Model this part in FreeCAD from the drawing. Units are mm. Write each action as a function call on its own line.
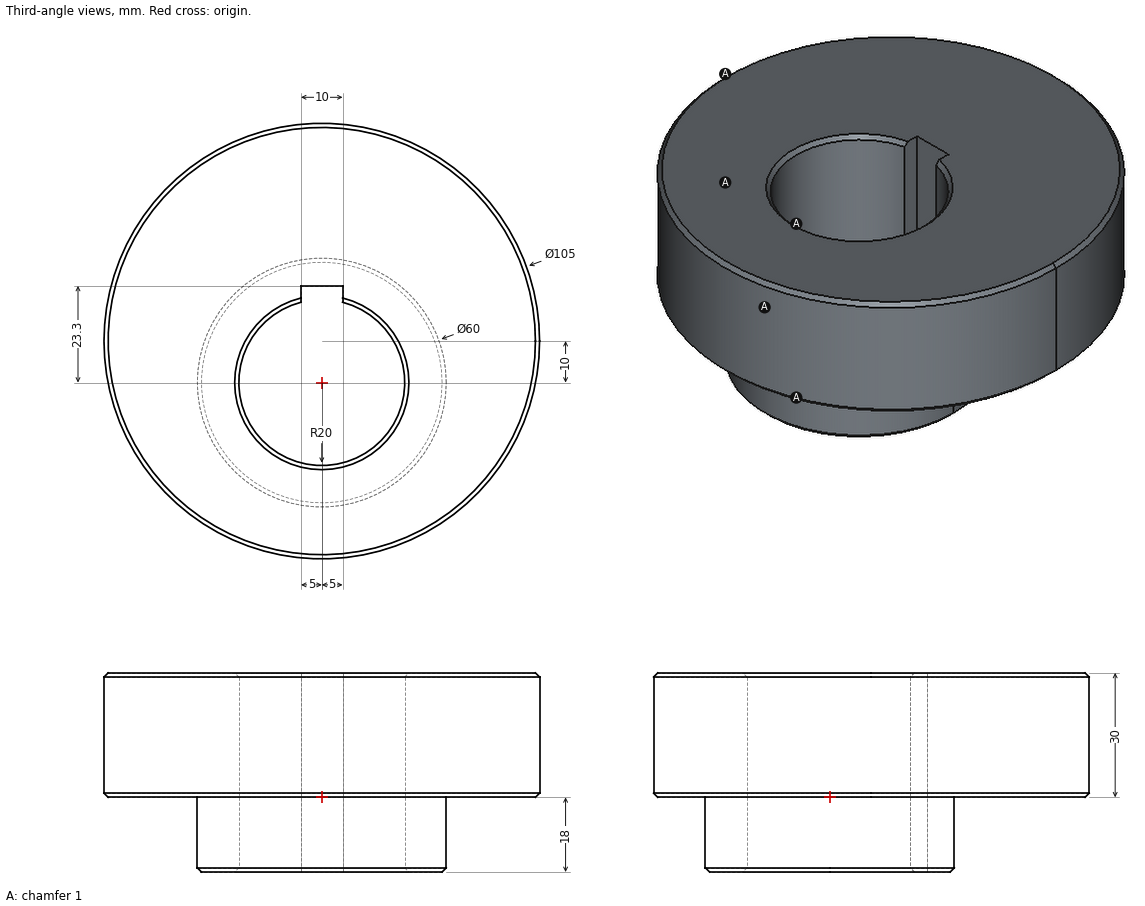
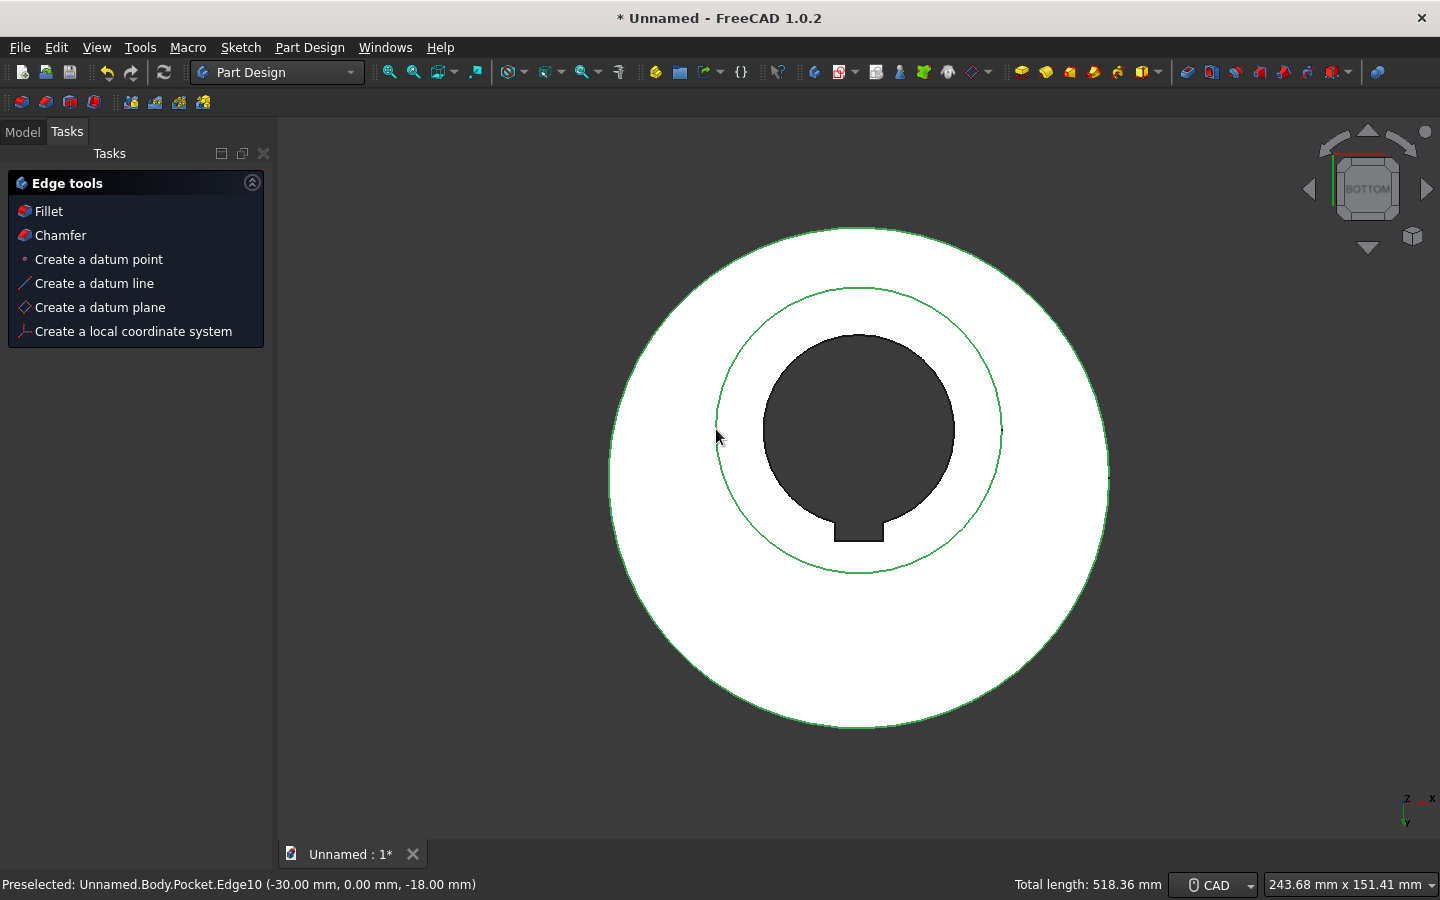
click(859, 334, ctrl)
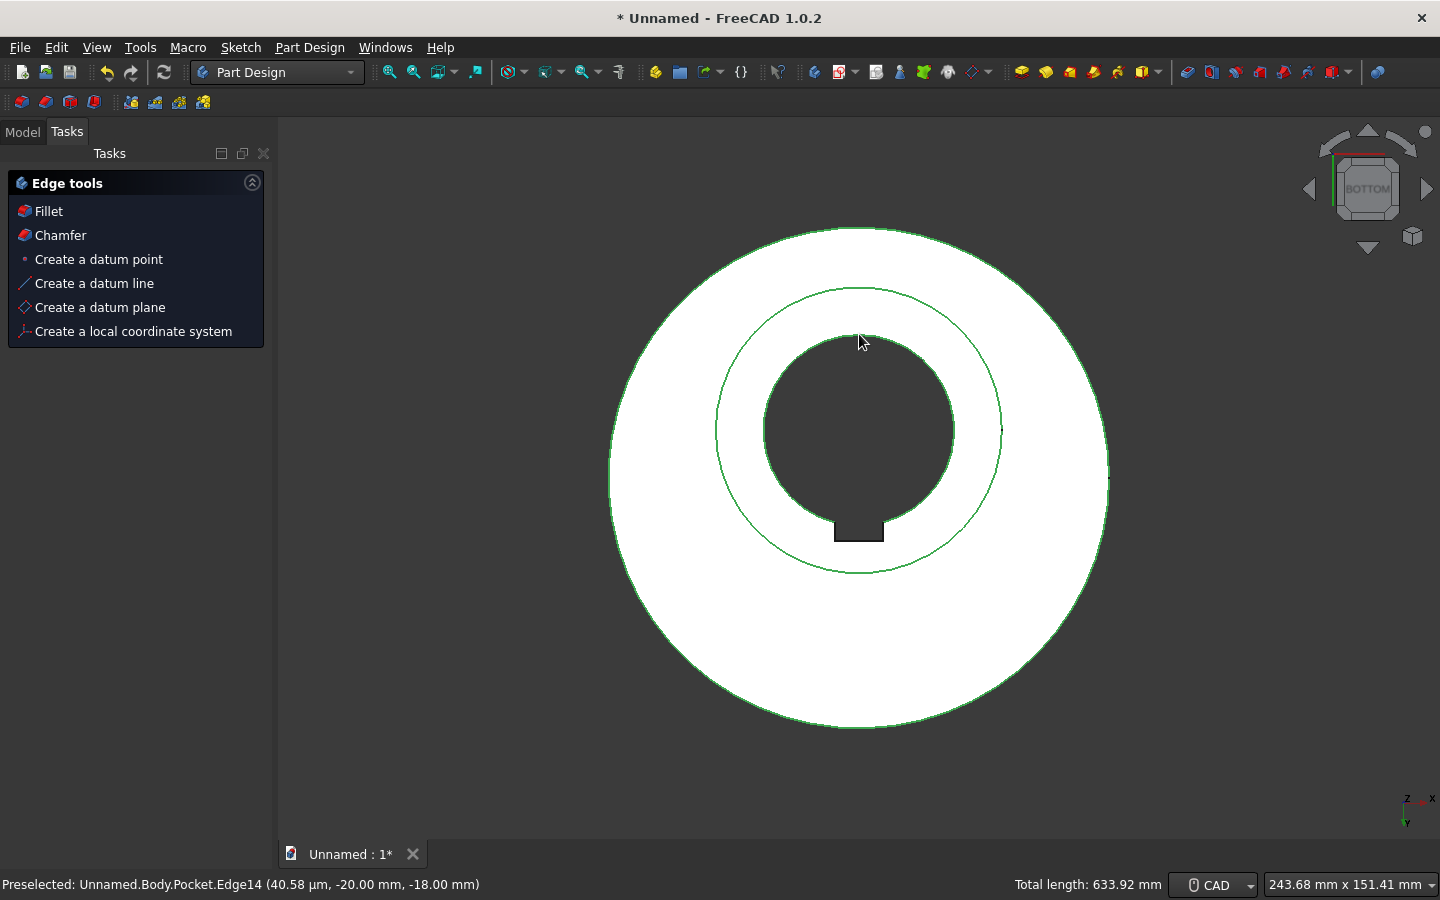
key(0)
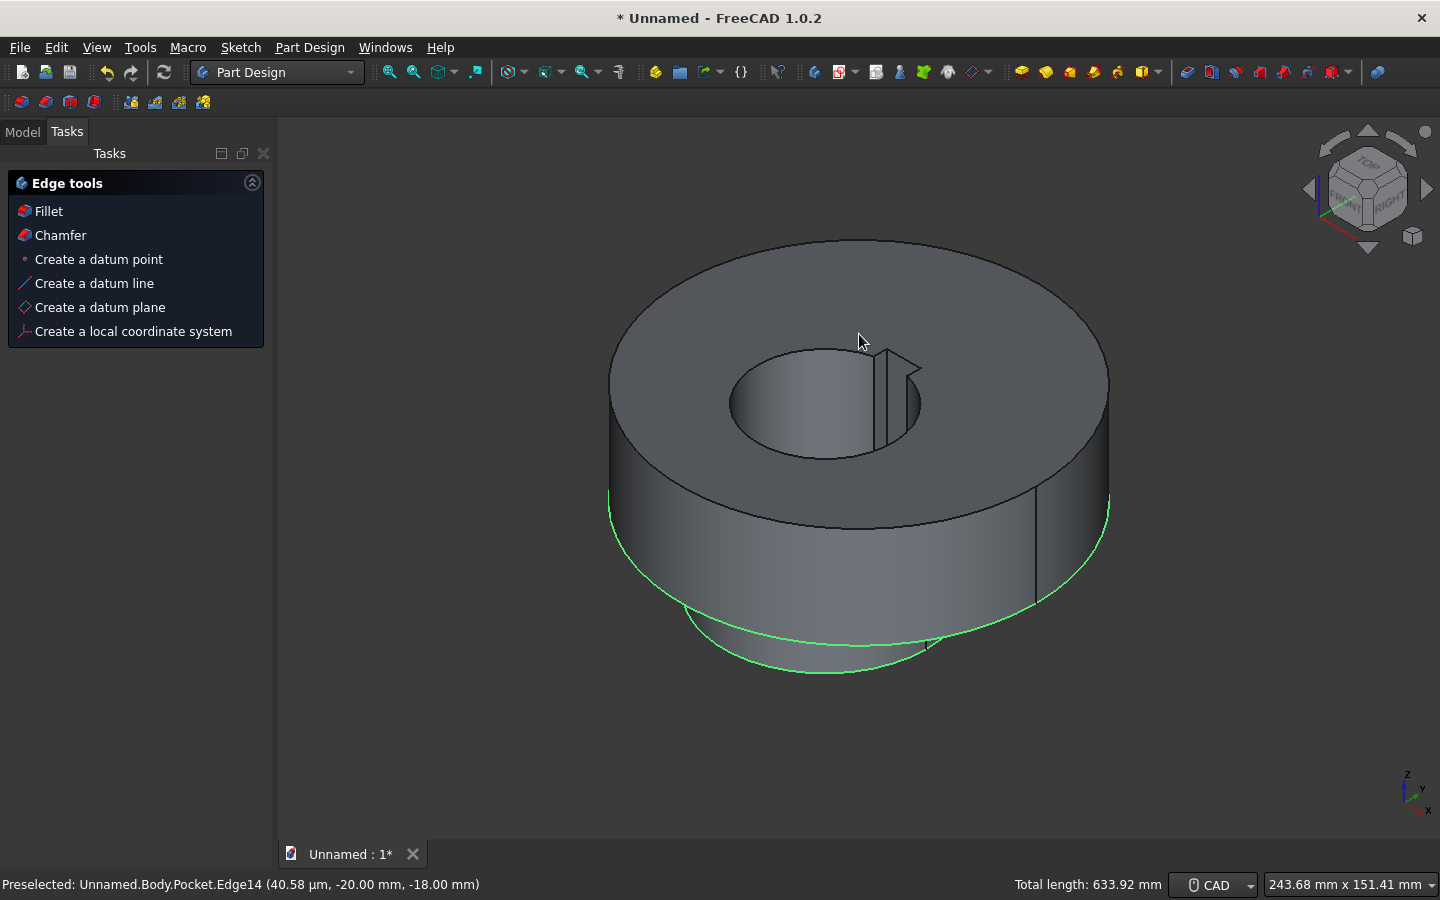
click(736, 383, ctrl)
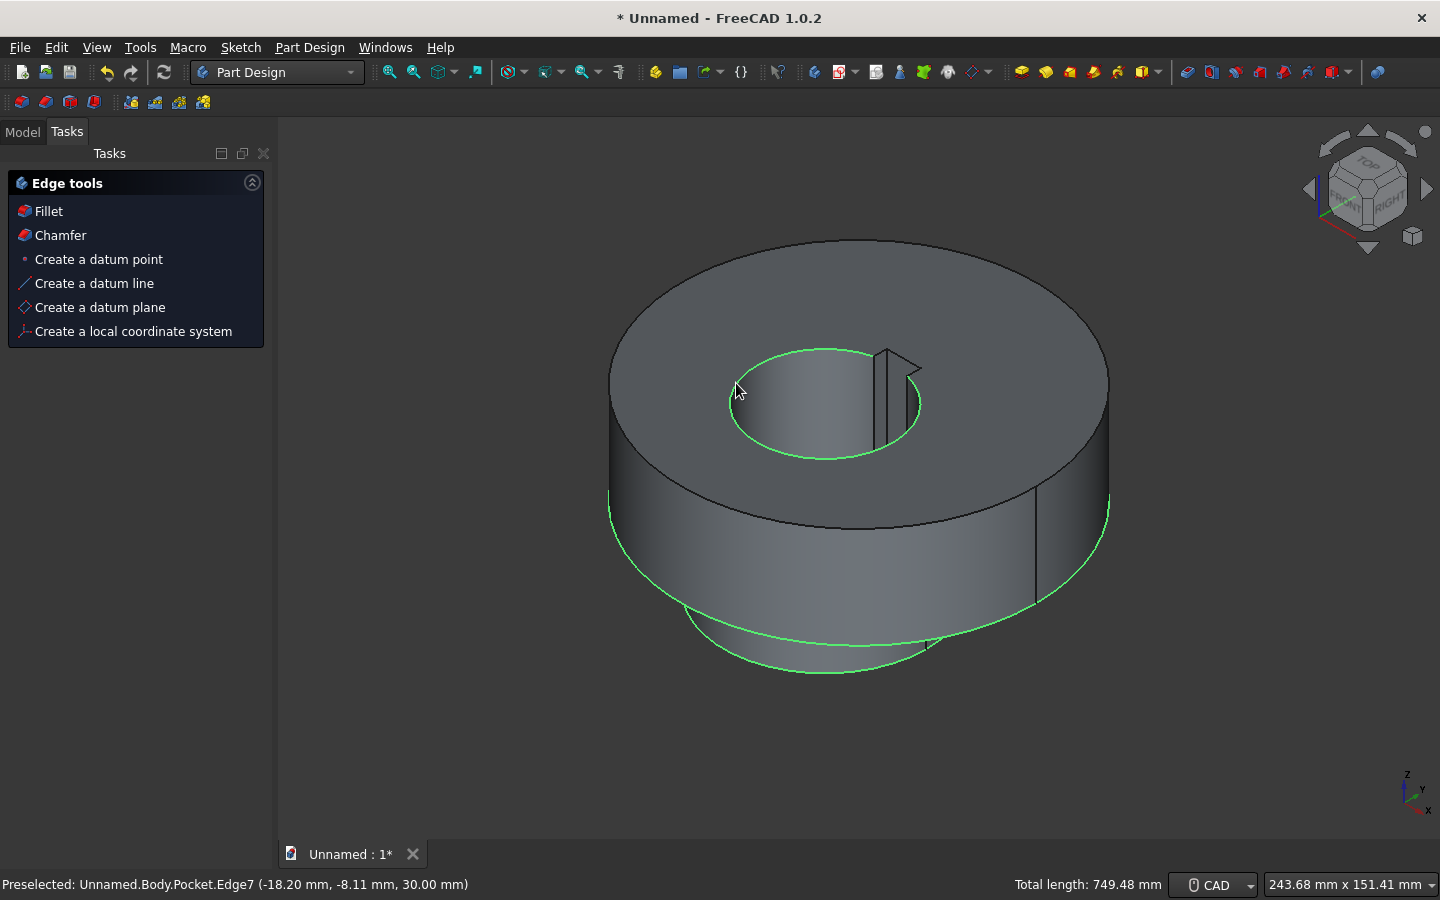
click(636, 449, ctrl)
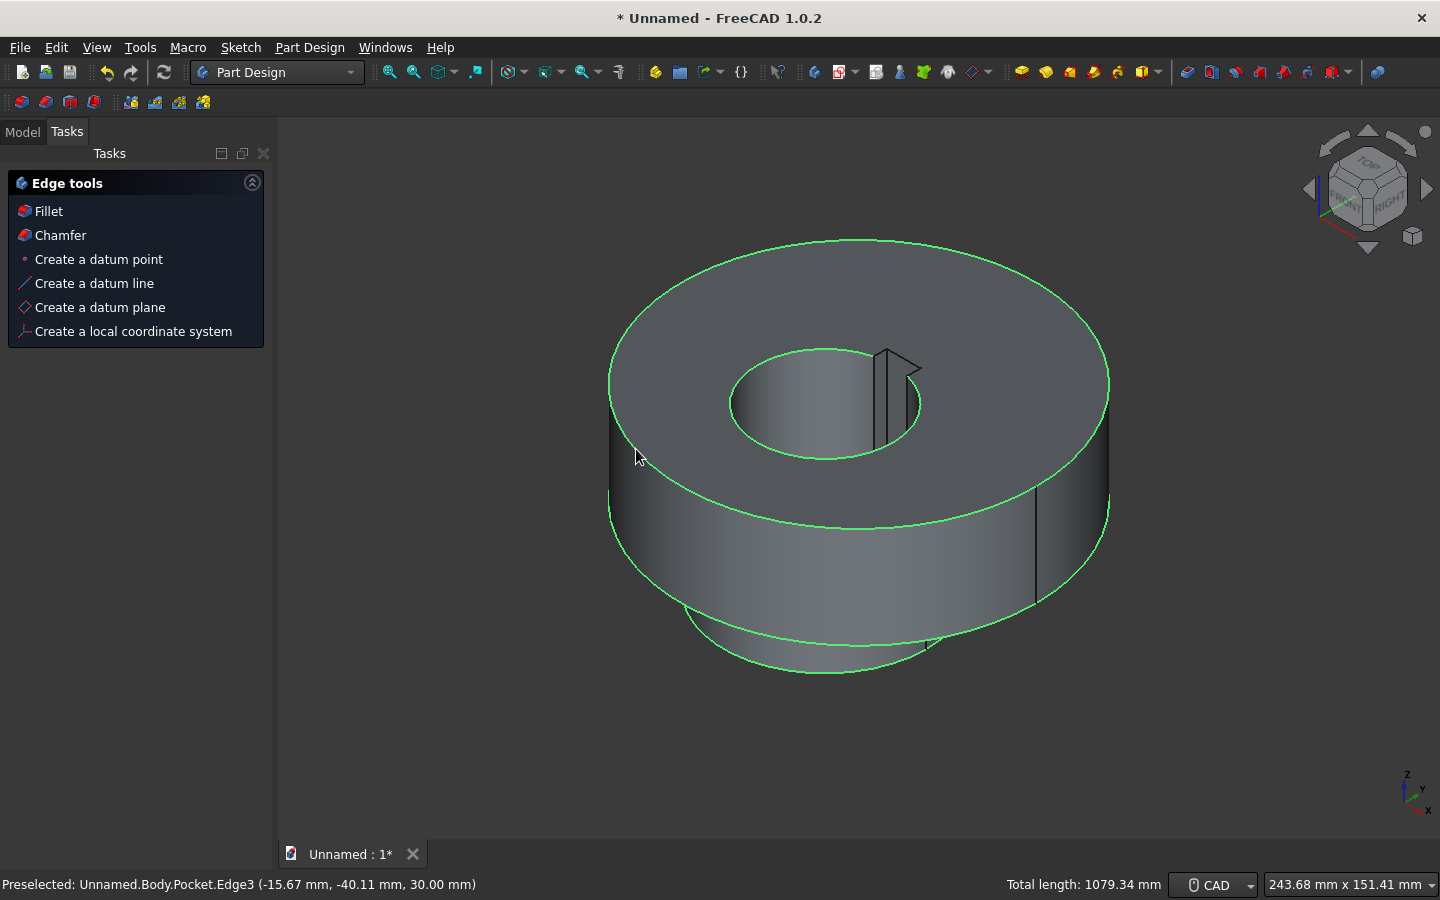
click(46, 102)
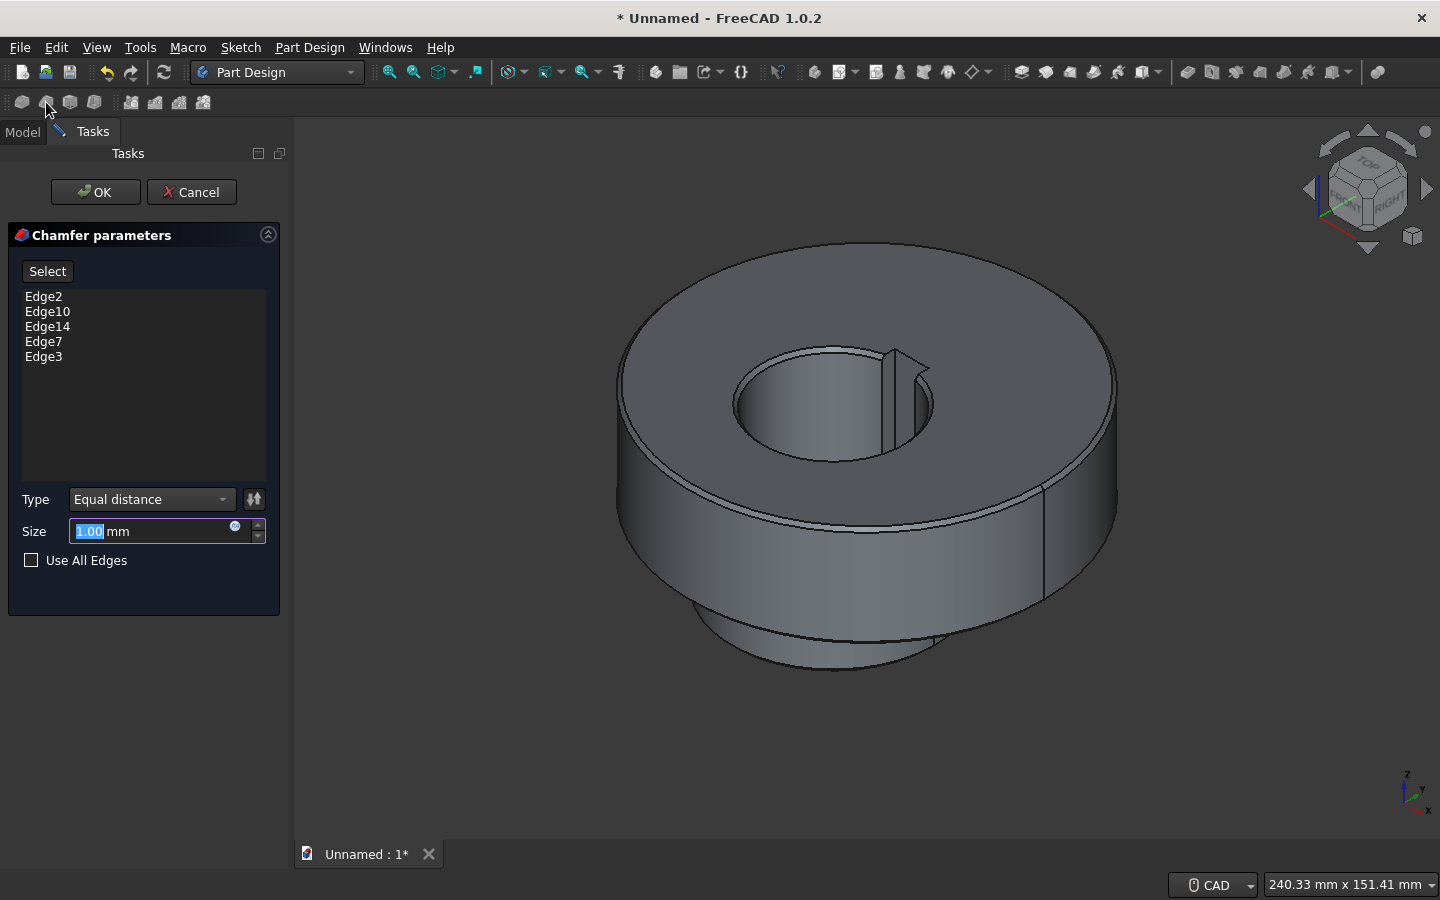
text(1)
key(Tab)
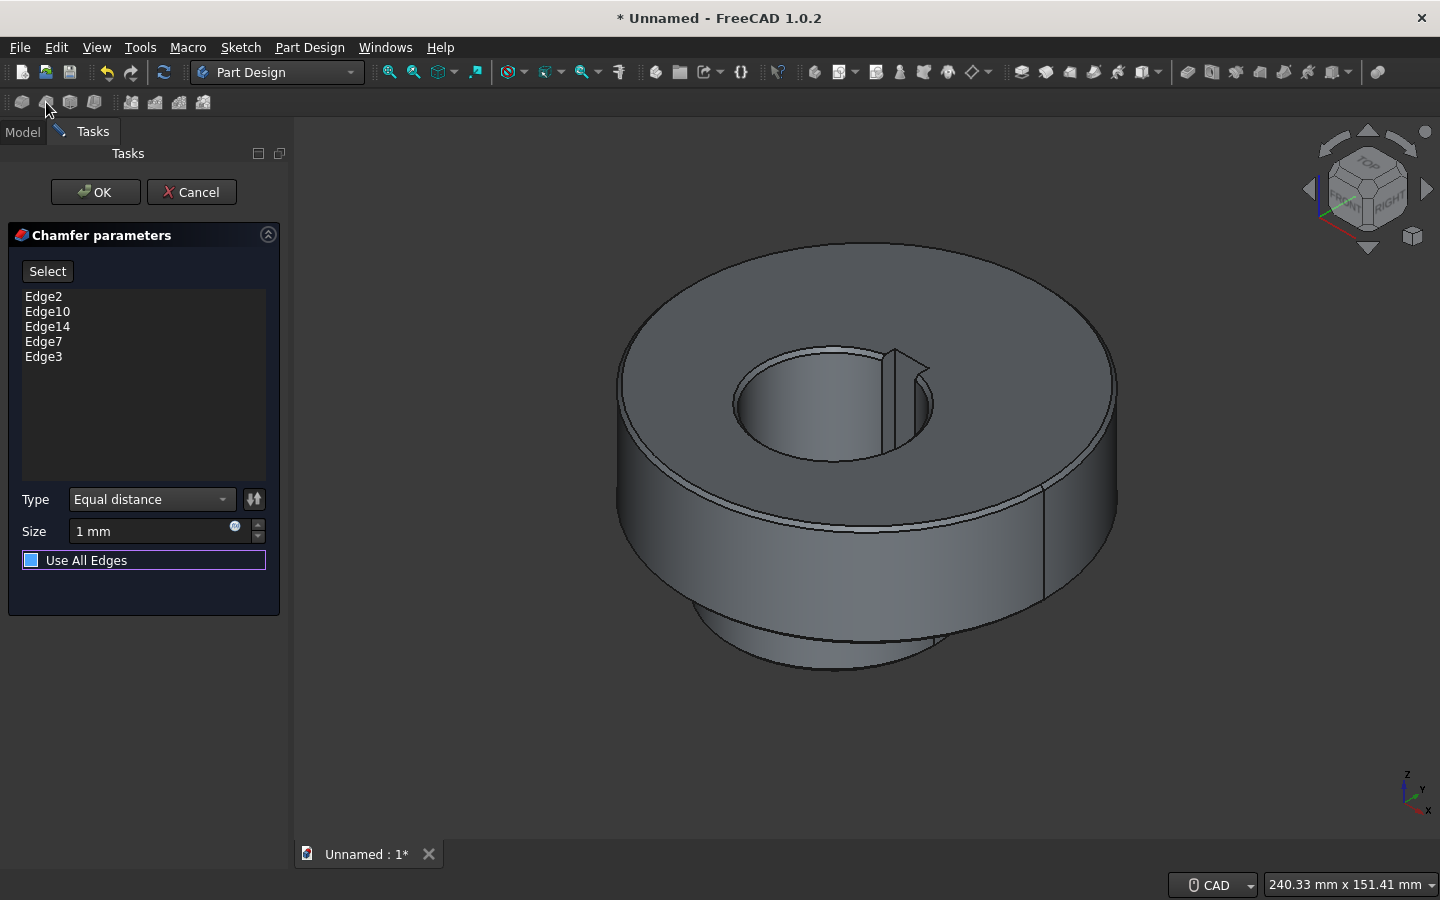
click(96, 192)